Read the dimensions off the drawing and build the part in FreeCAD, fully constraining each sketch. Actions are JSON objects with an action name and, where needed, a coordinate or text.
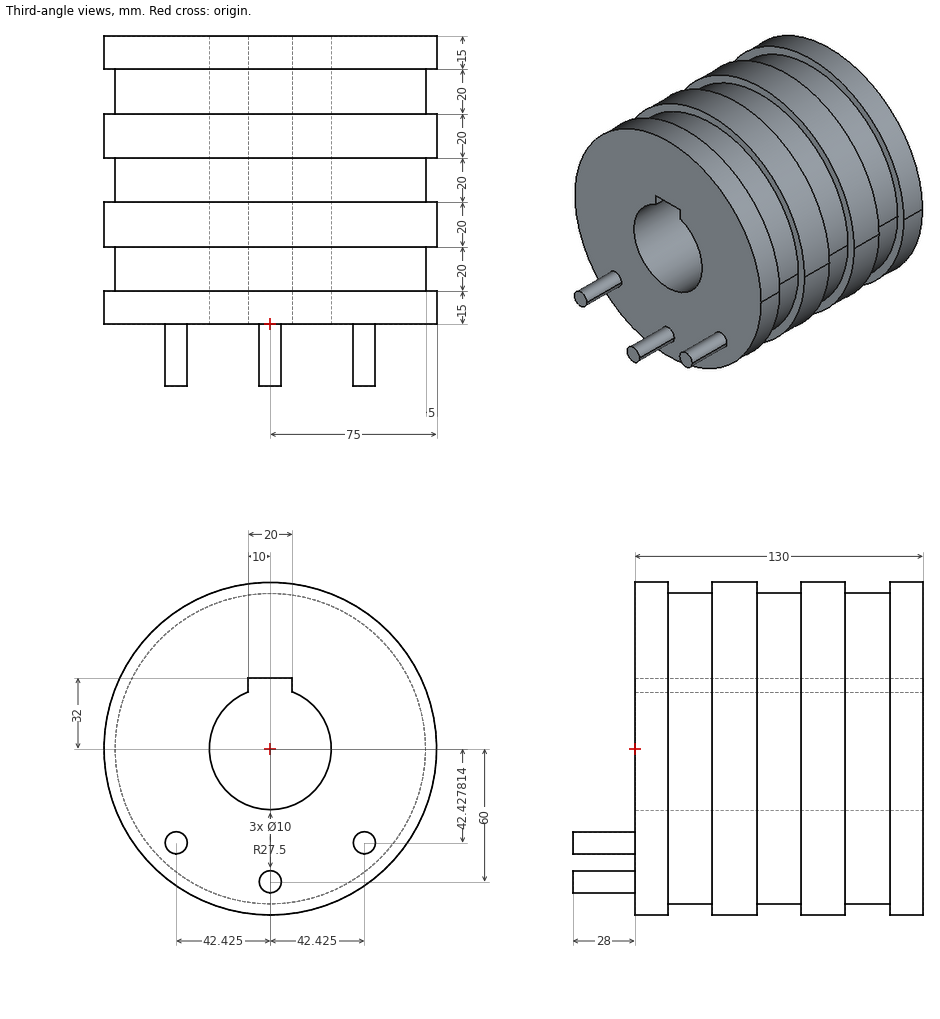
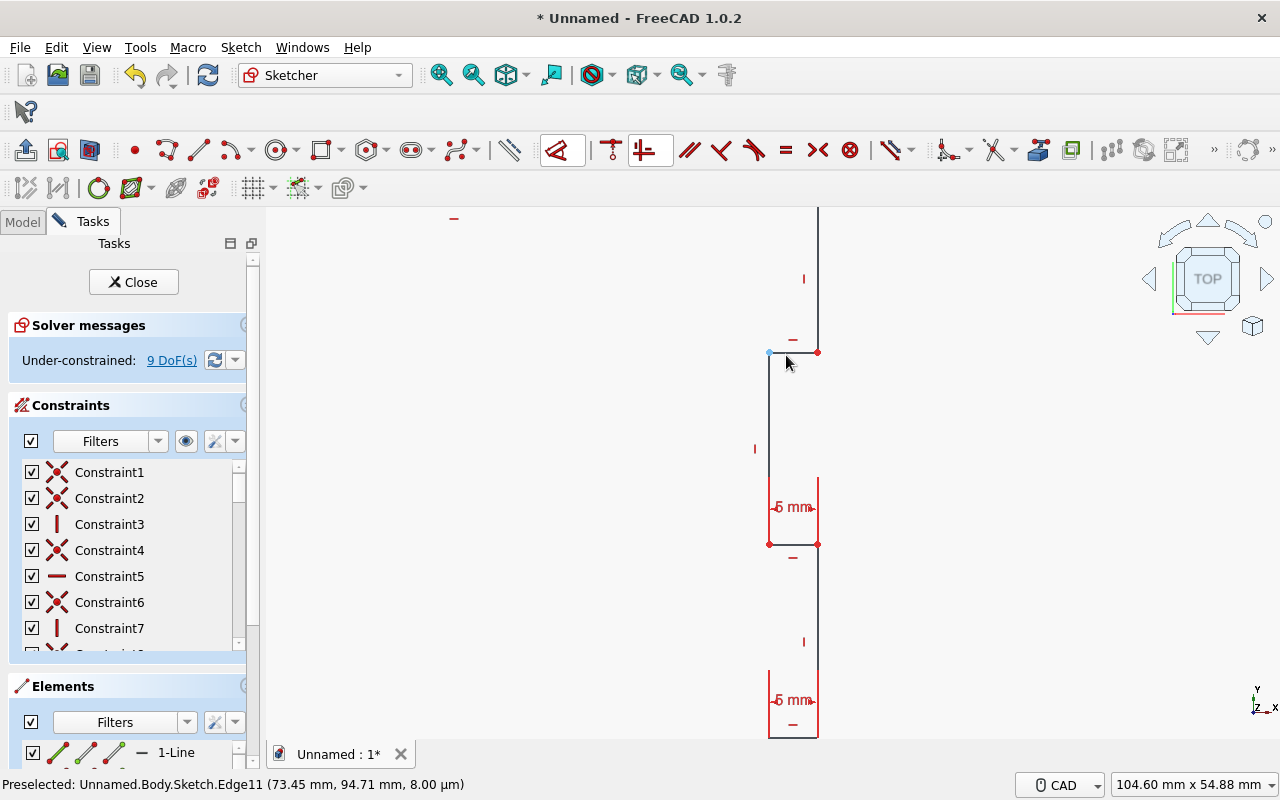
{"action": "left_click", "coordinate": [784, 353]}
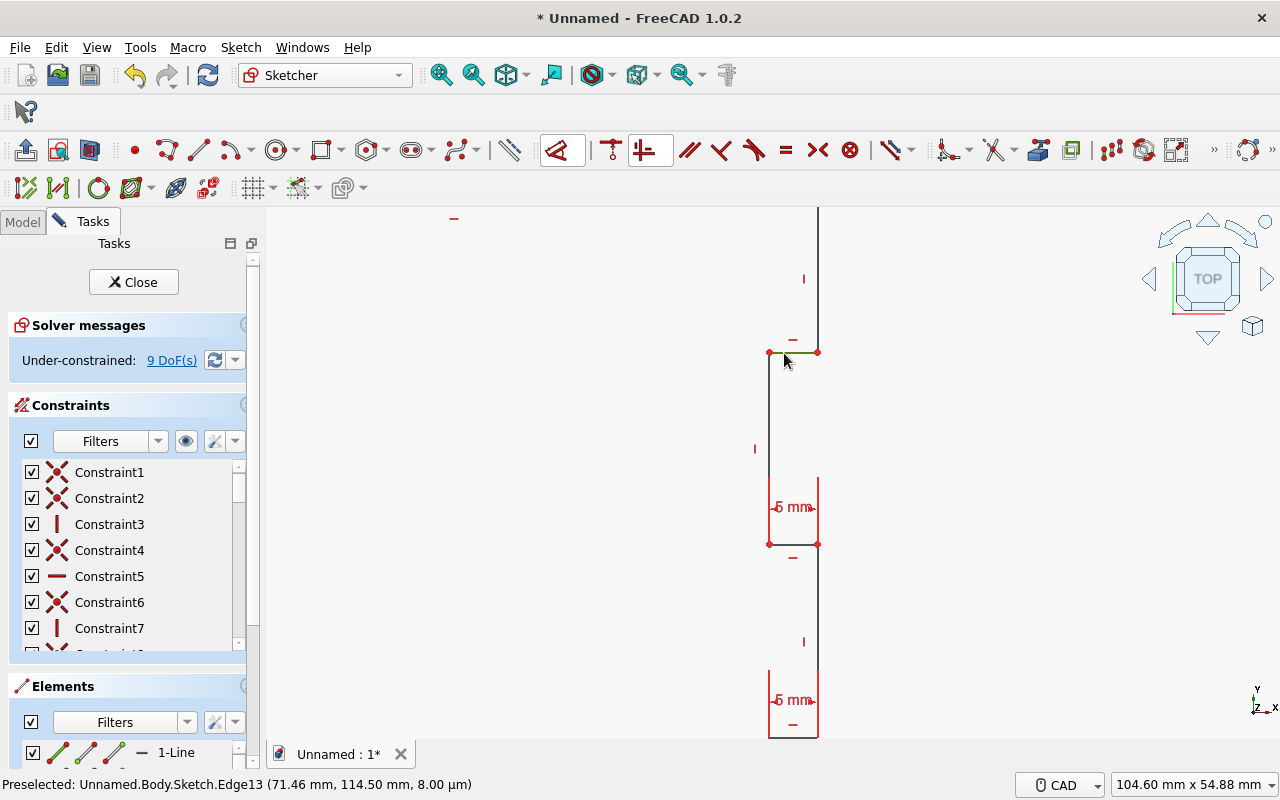
{"action": "left_click", "coordinate": [580, 150]}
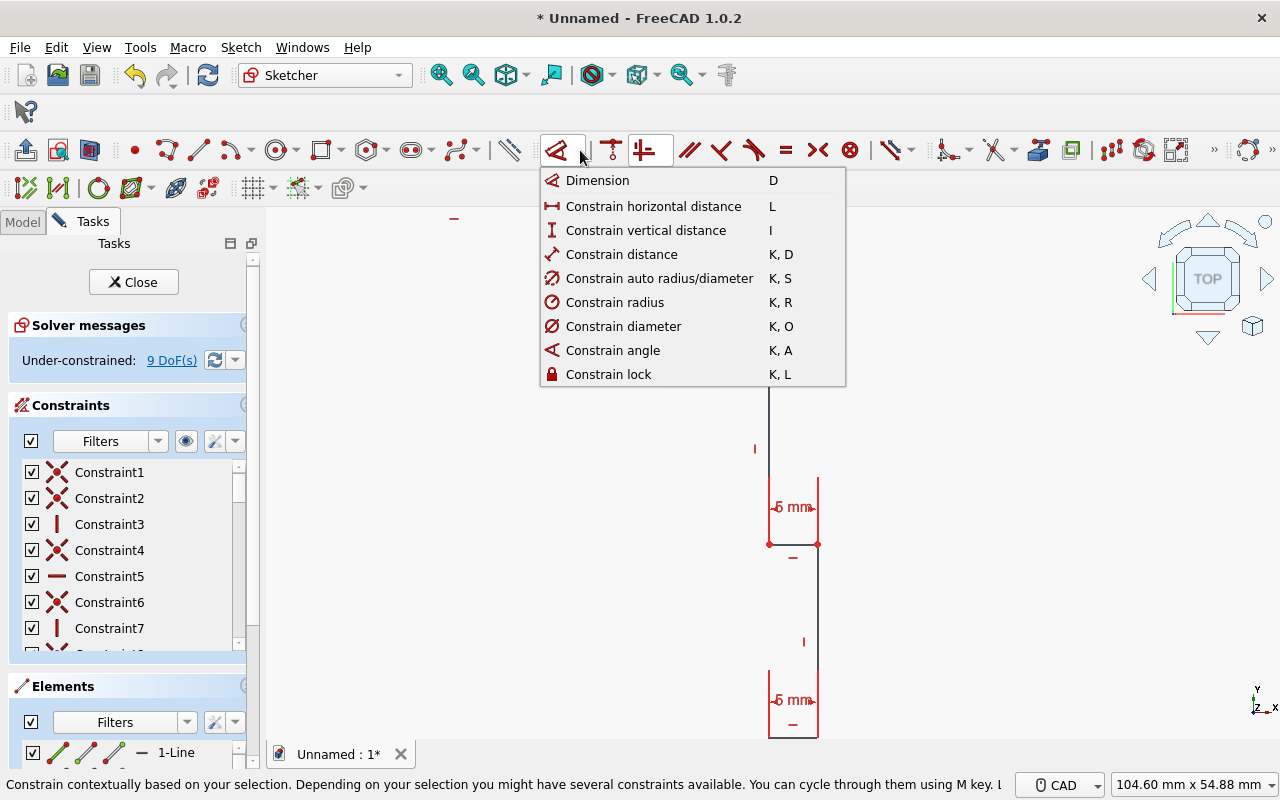
{"action": "left_click", "coordinate": [693, 206]}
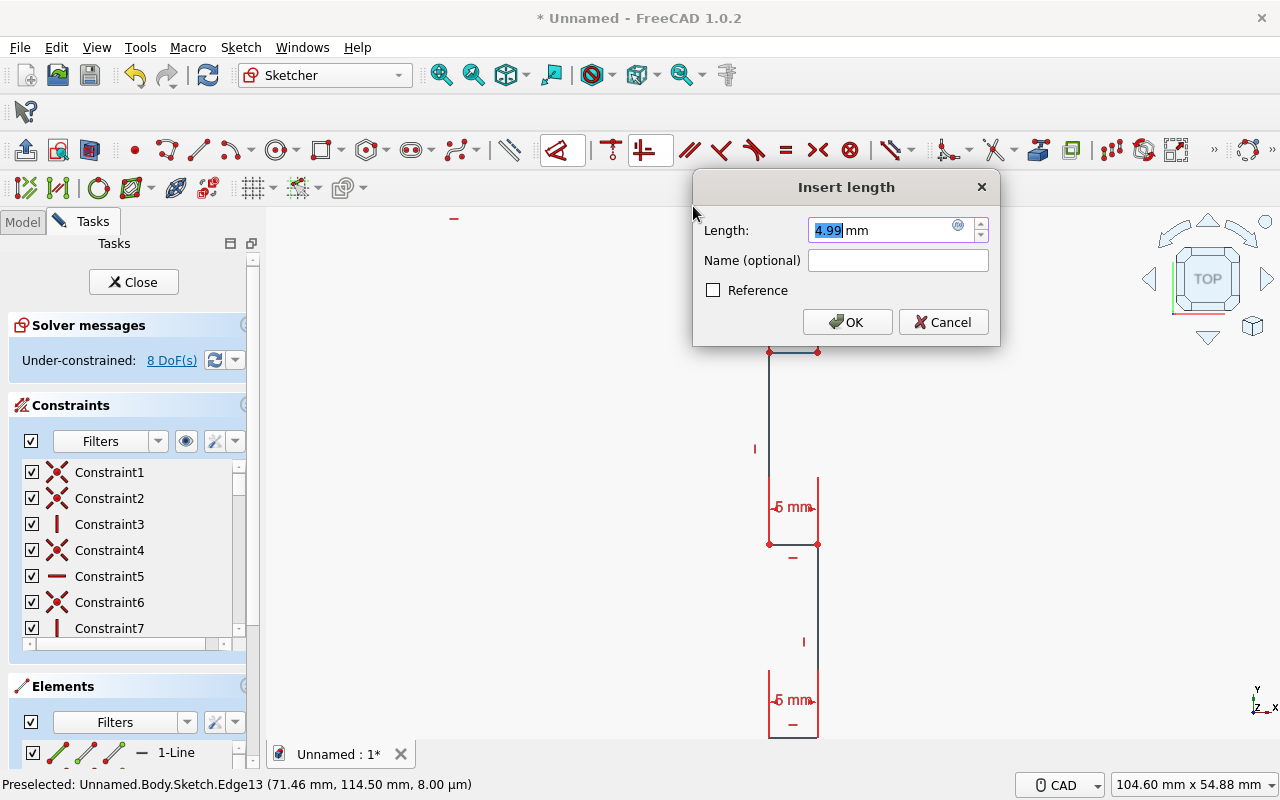
{"action": "type", "text": "5"}
{"action": "key", "text": "Return"}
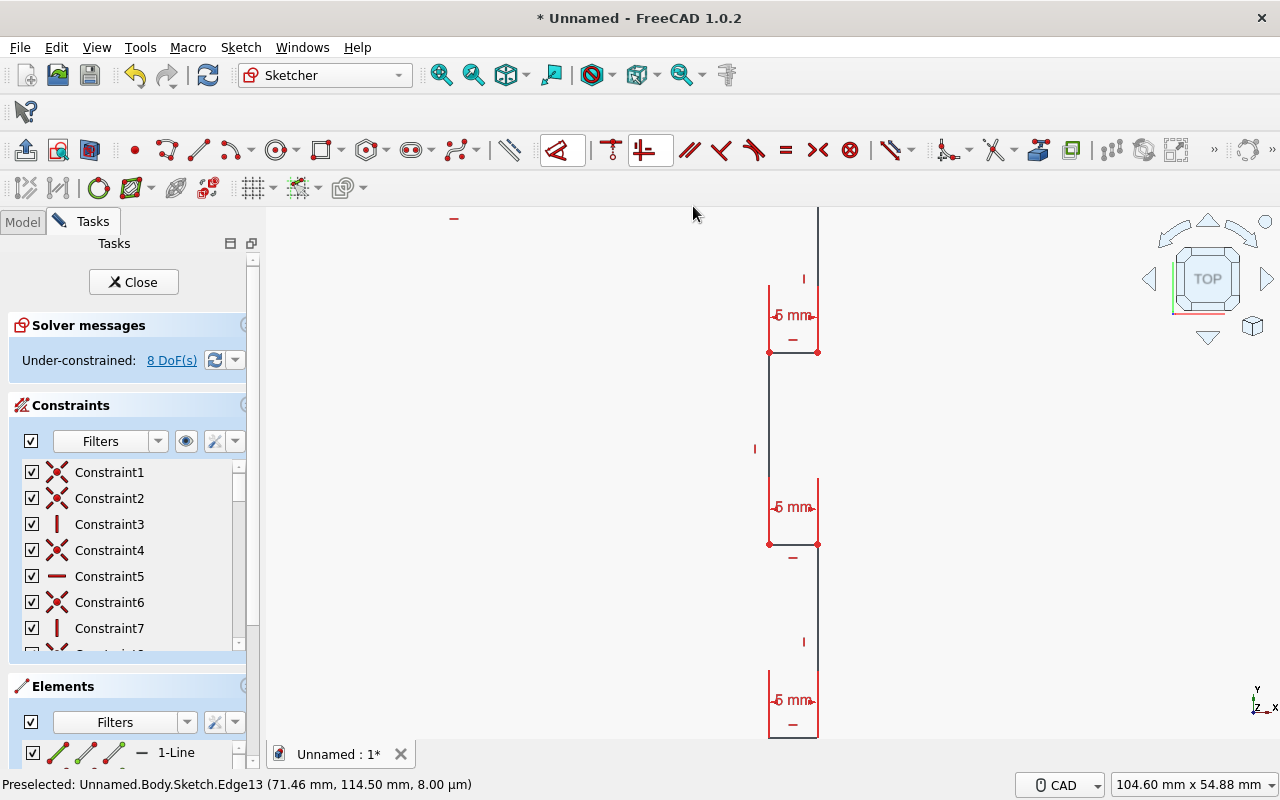
{"action": "scroll", "coordinate": [786, 355], "scroll_direction": "down", "scroll_amount": 7}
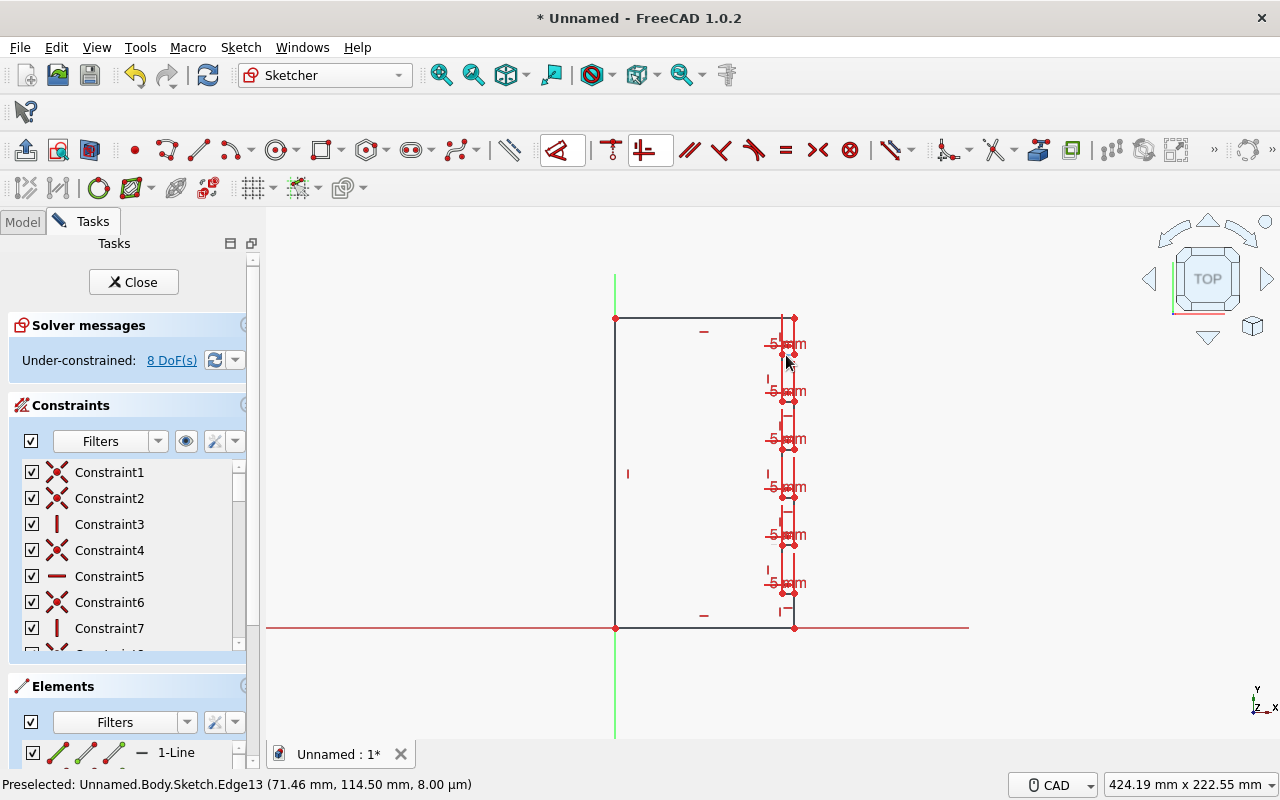
{"action": "left_click", "coordinate": [669, 628]}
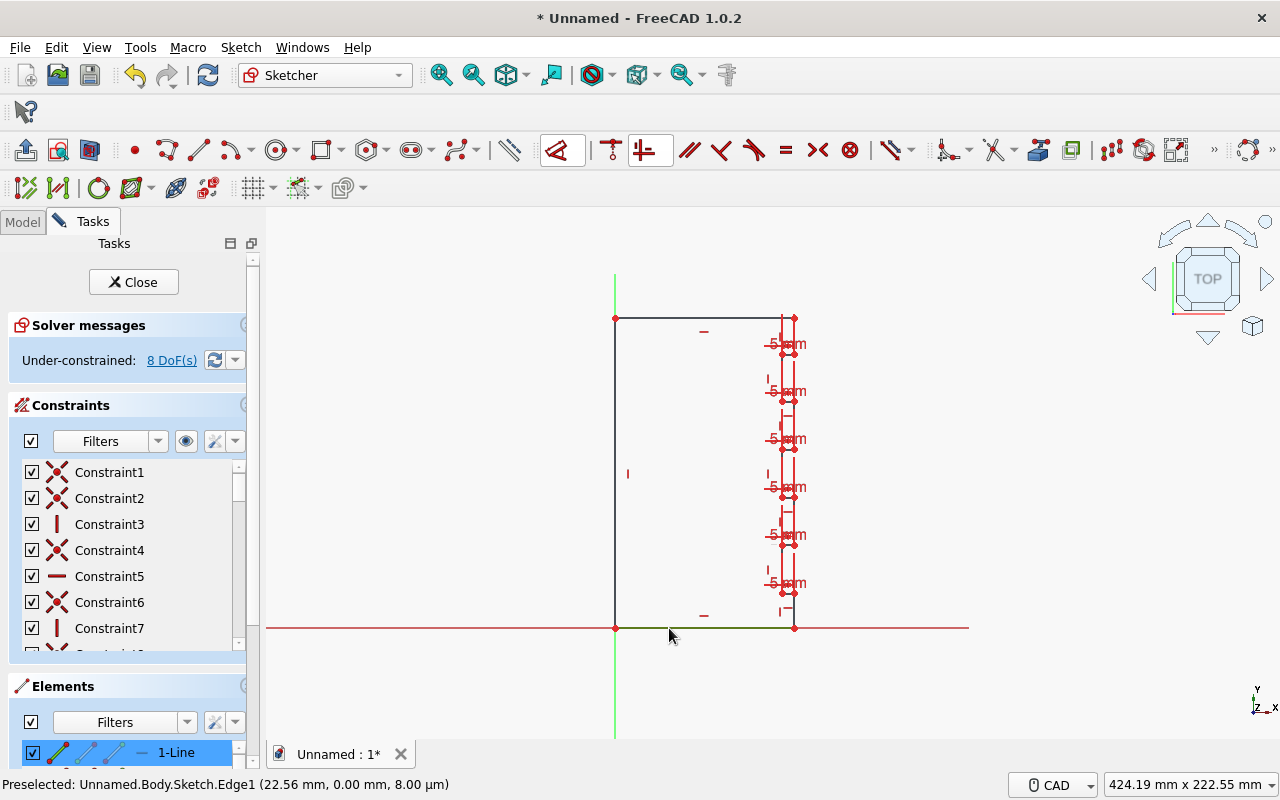
{"action": "key", "text": "l"}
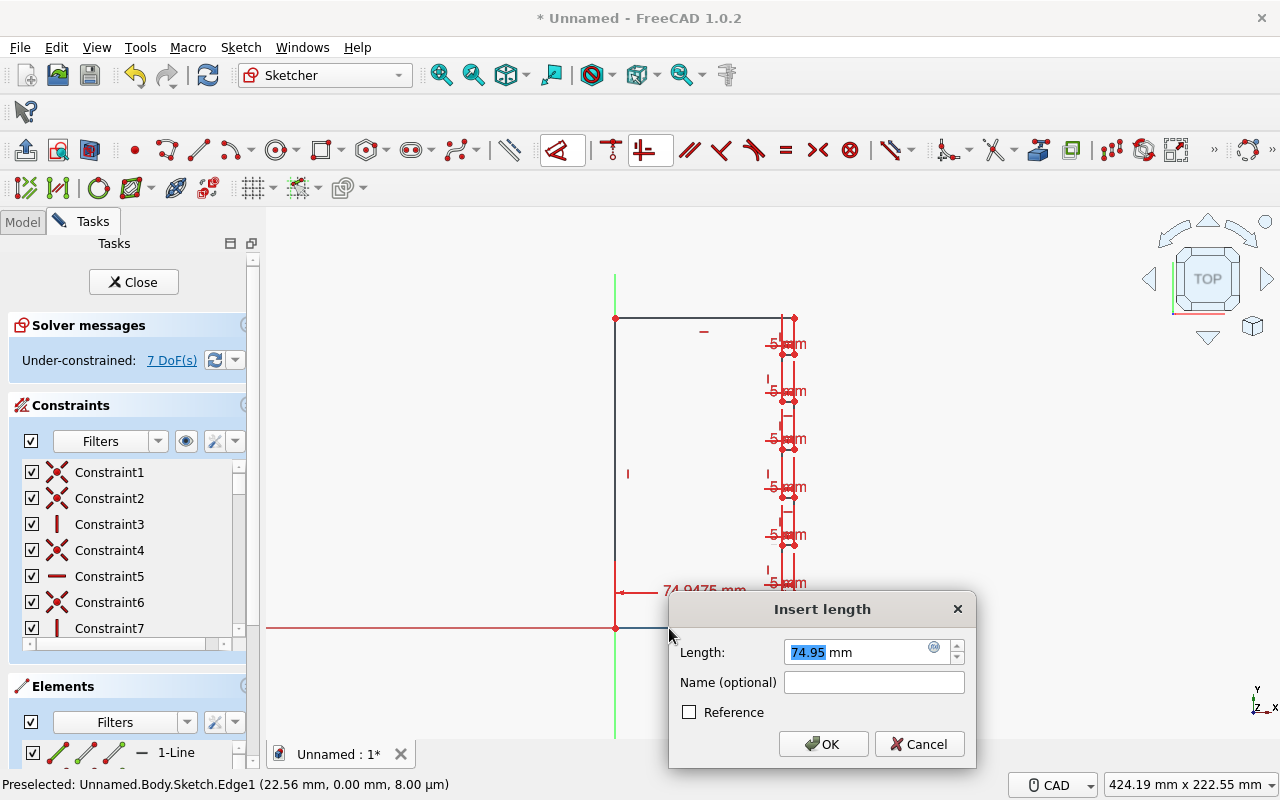
{"action": "type", "text": "75"}
{"action": "key", "text": "Return"}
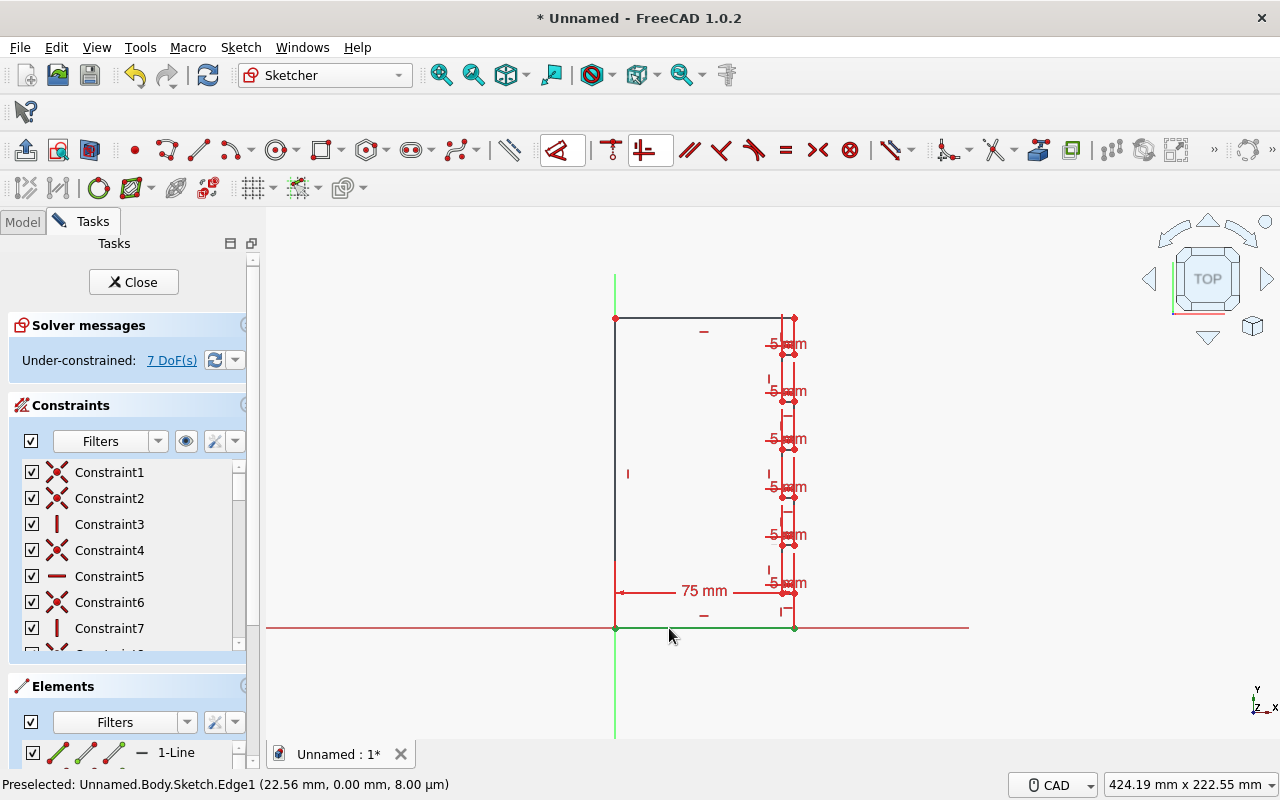
{"action": "scroll", "coordinate": [794, 618], "scroll_direction": "up", "scroll_amount": 2}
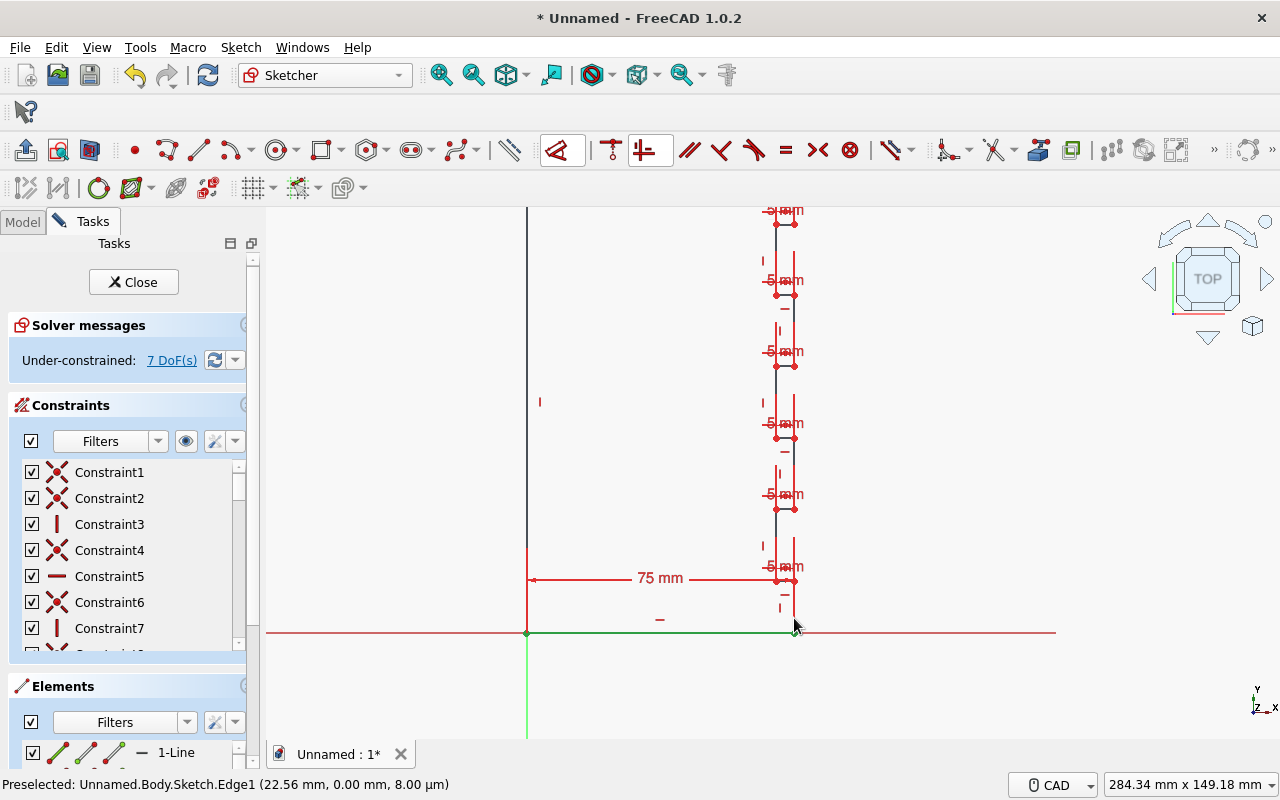
{"action": "left_click", "coordinate": [794, 618]}